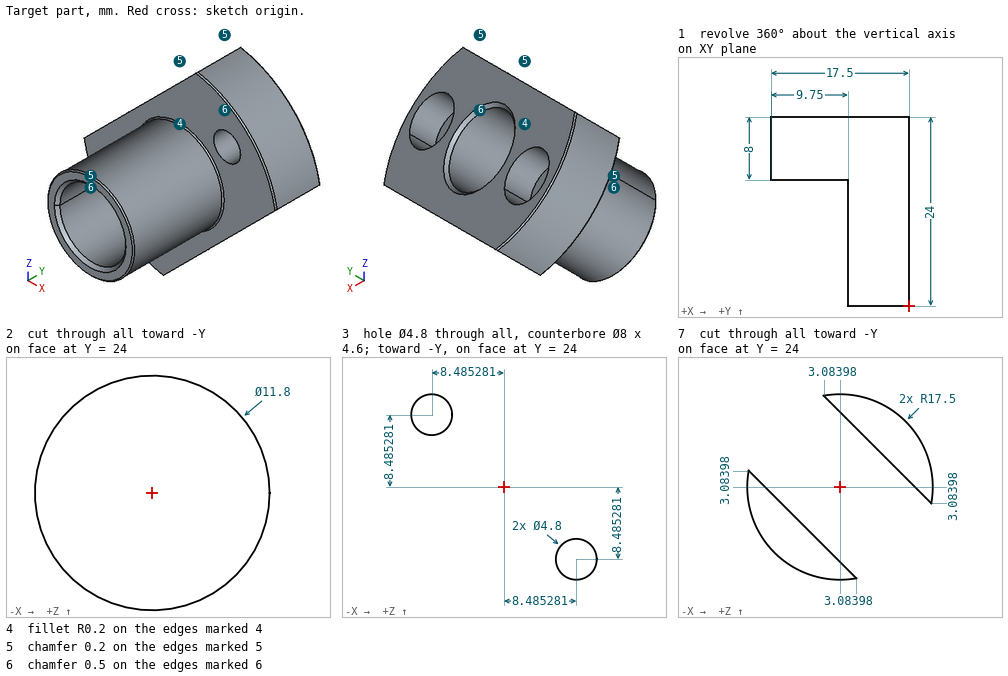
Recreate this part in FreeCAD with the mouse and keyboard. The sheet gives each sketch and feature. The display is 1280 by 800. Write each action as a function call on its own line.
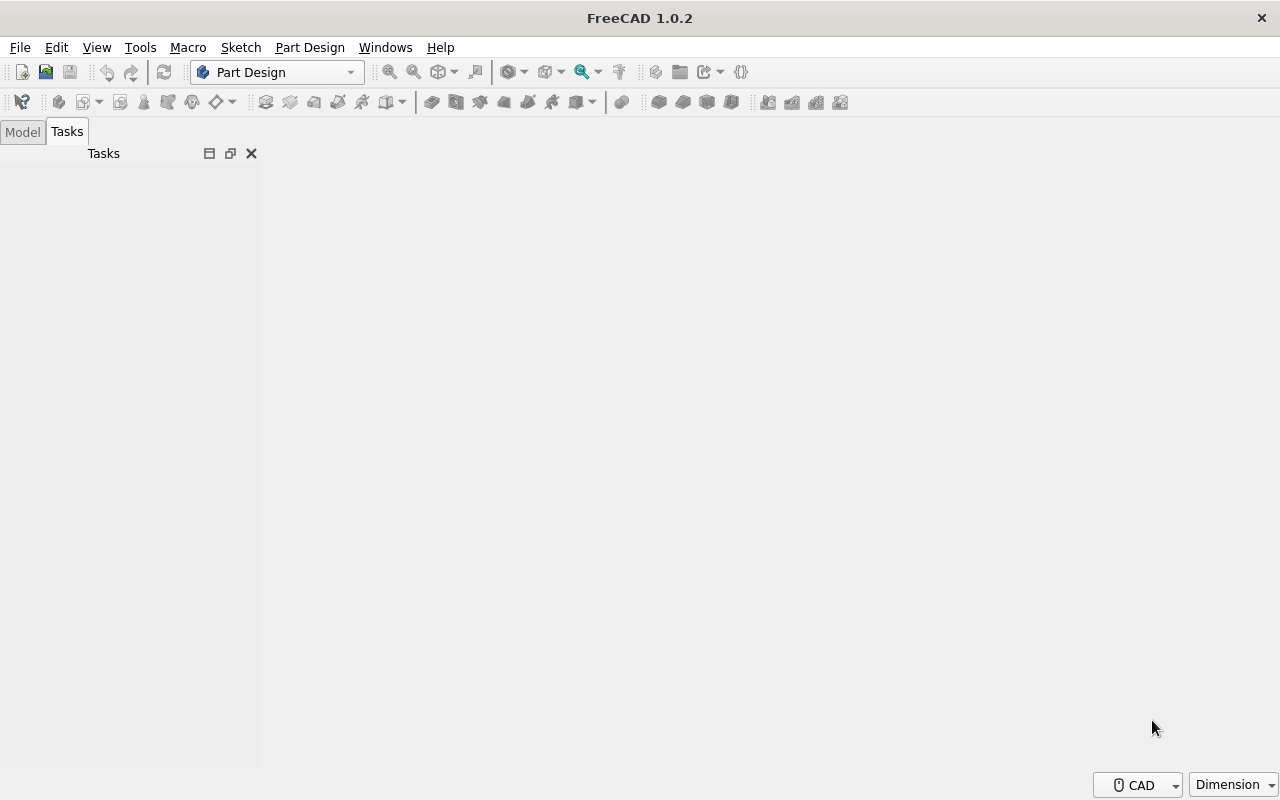
key(ctrl+n)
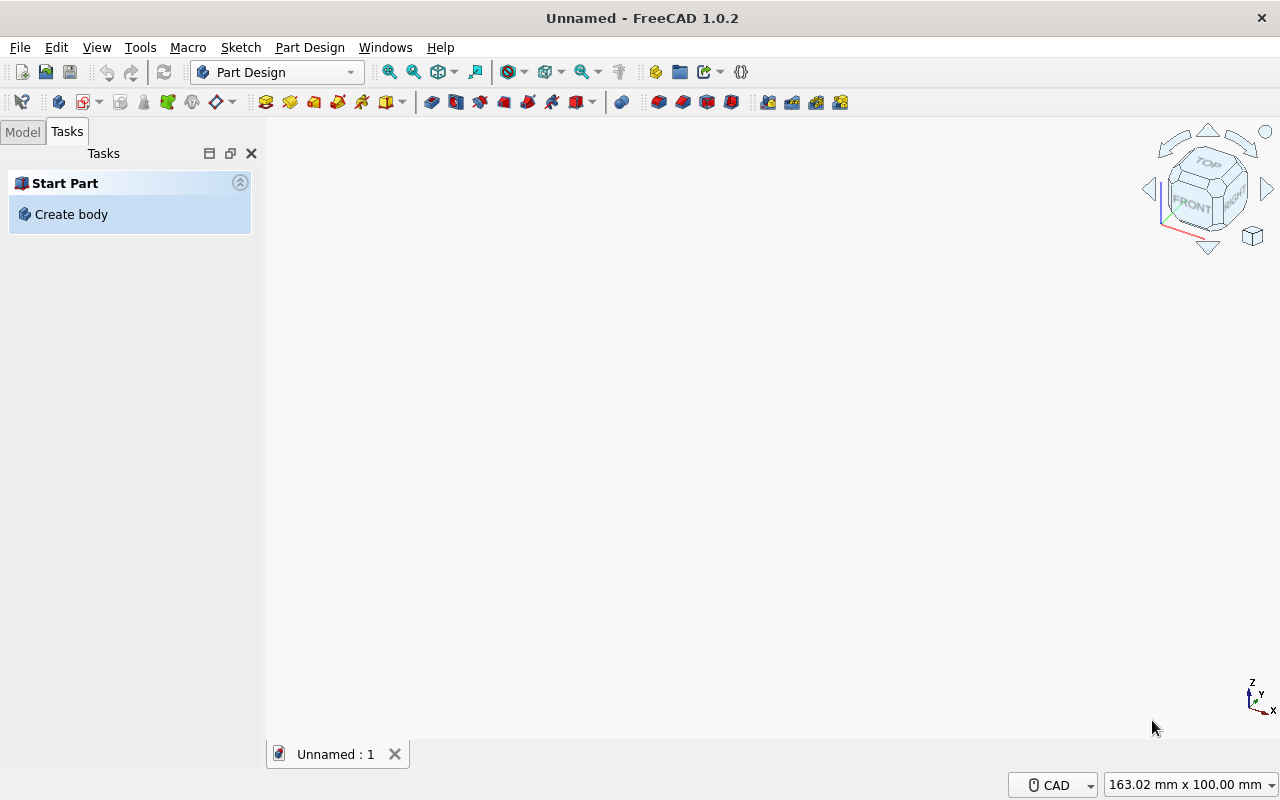
click(84, 102)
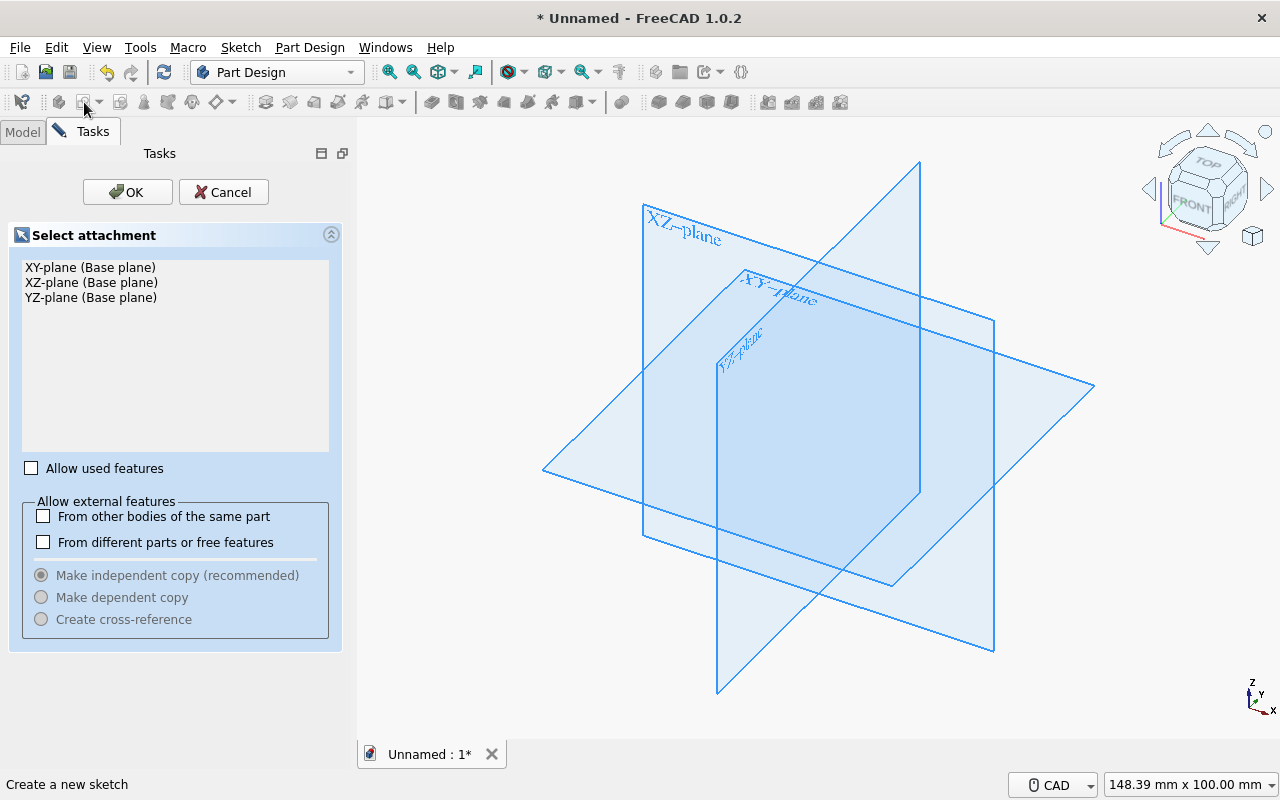
click(82, 268)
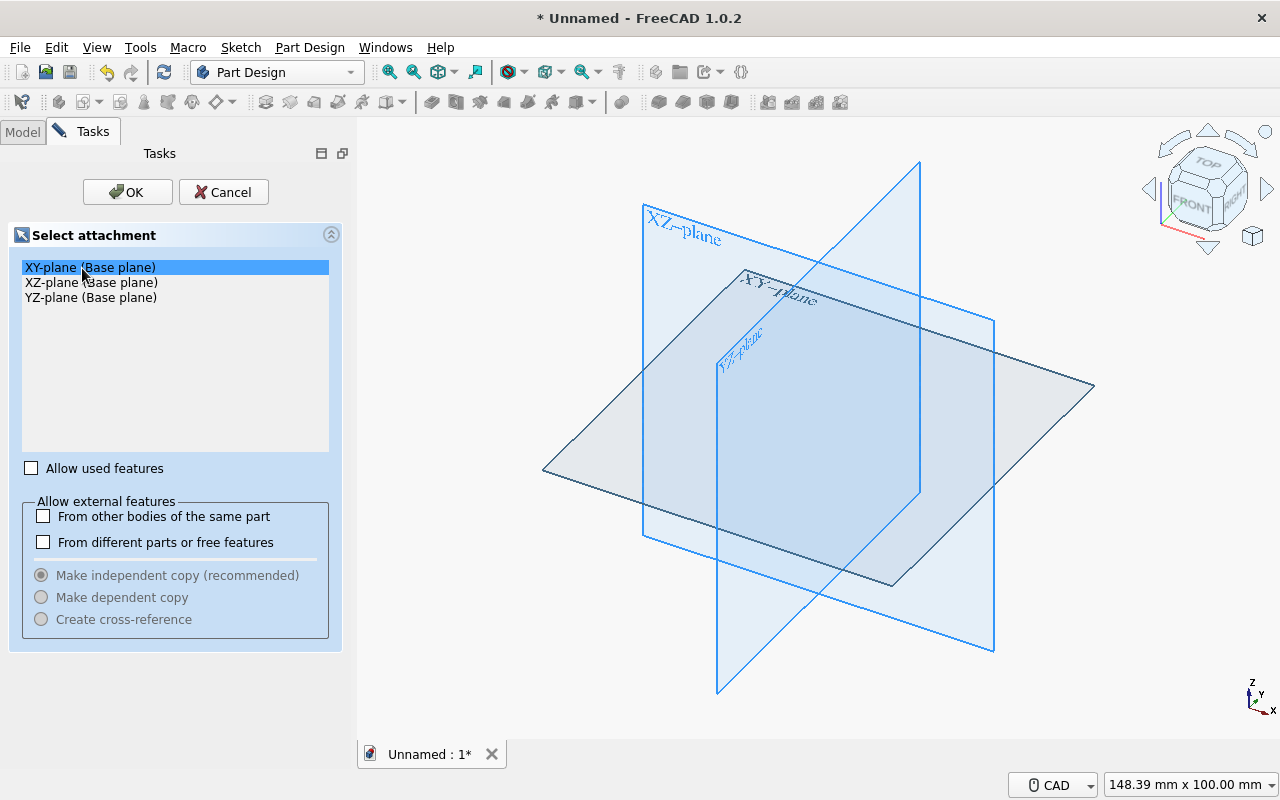
click(128, 192)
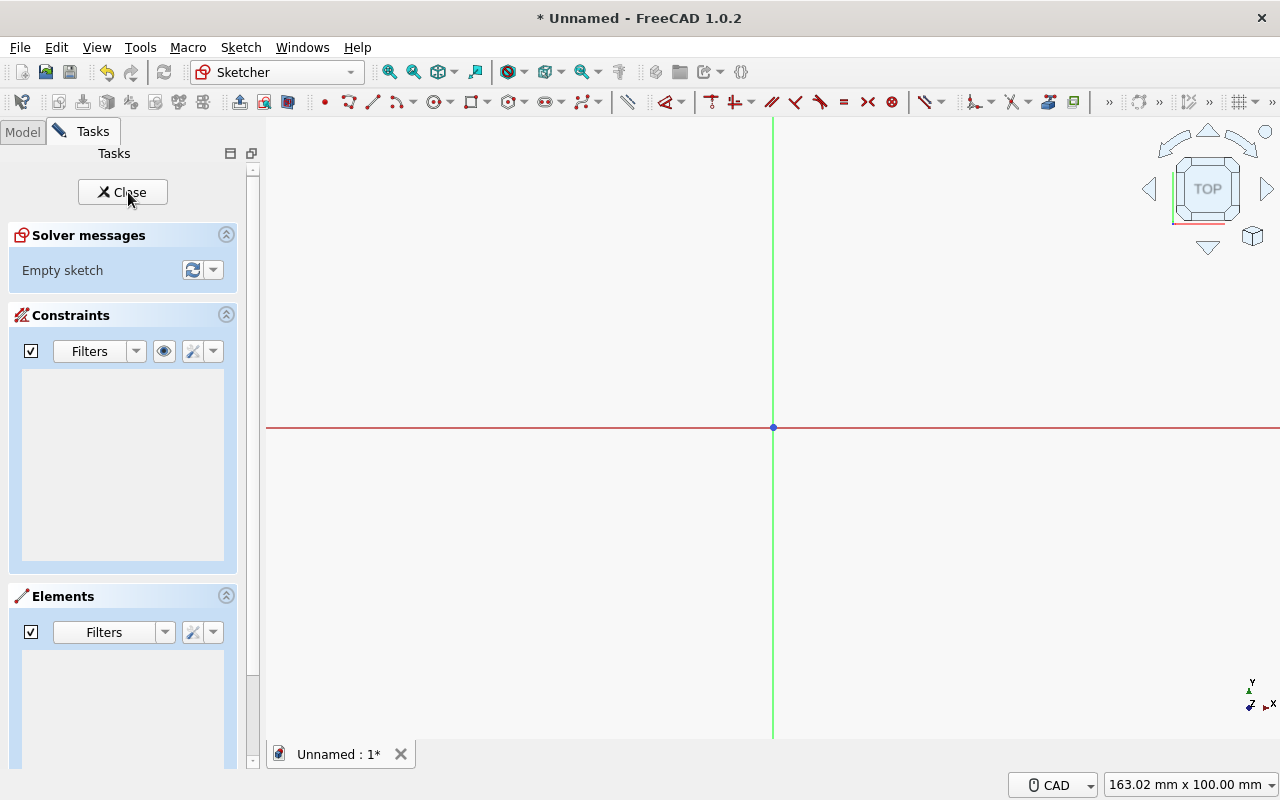
scroll(727, 310, up, 5)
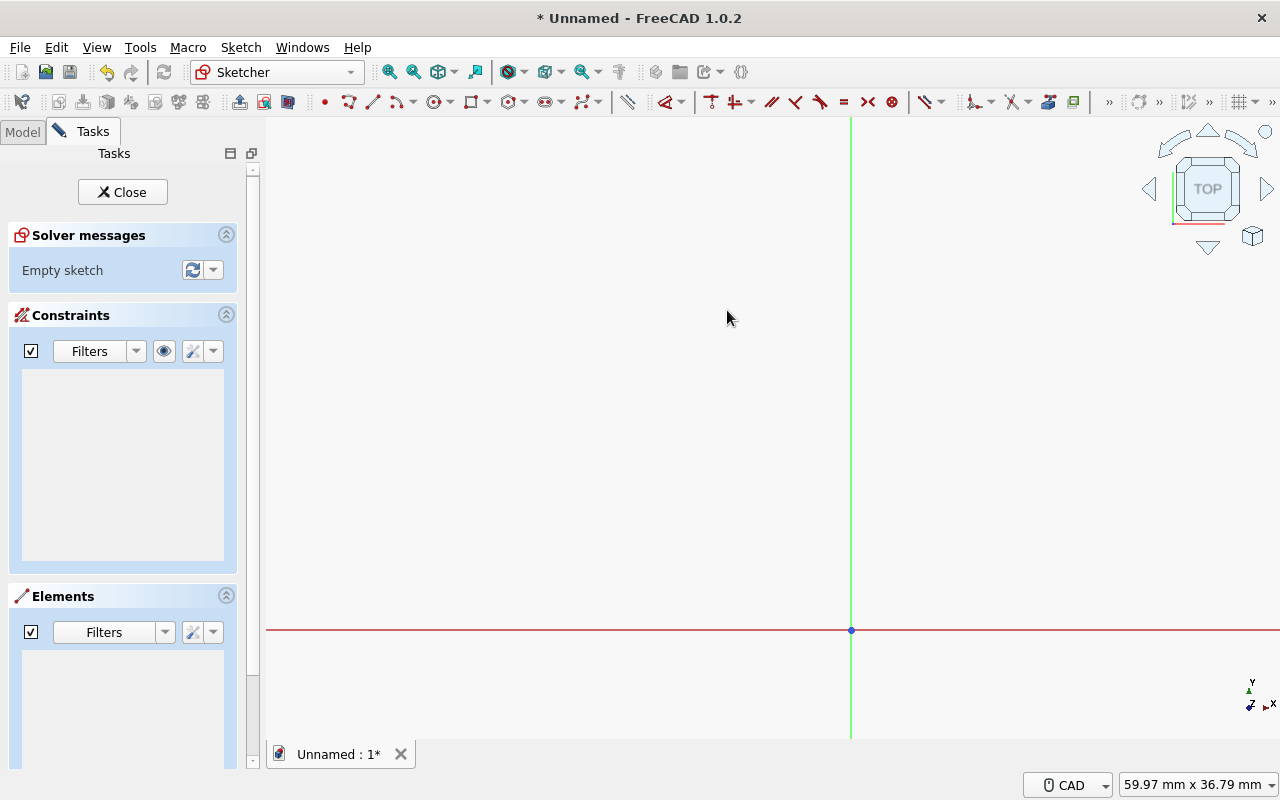
key(g)
key(m)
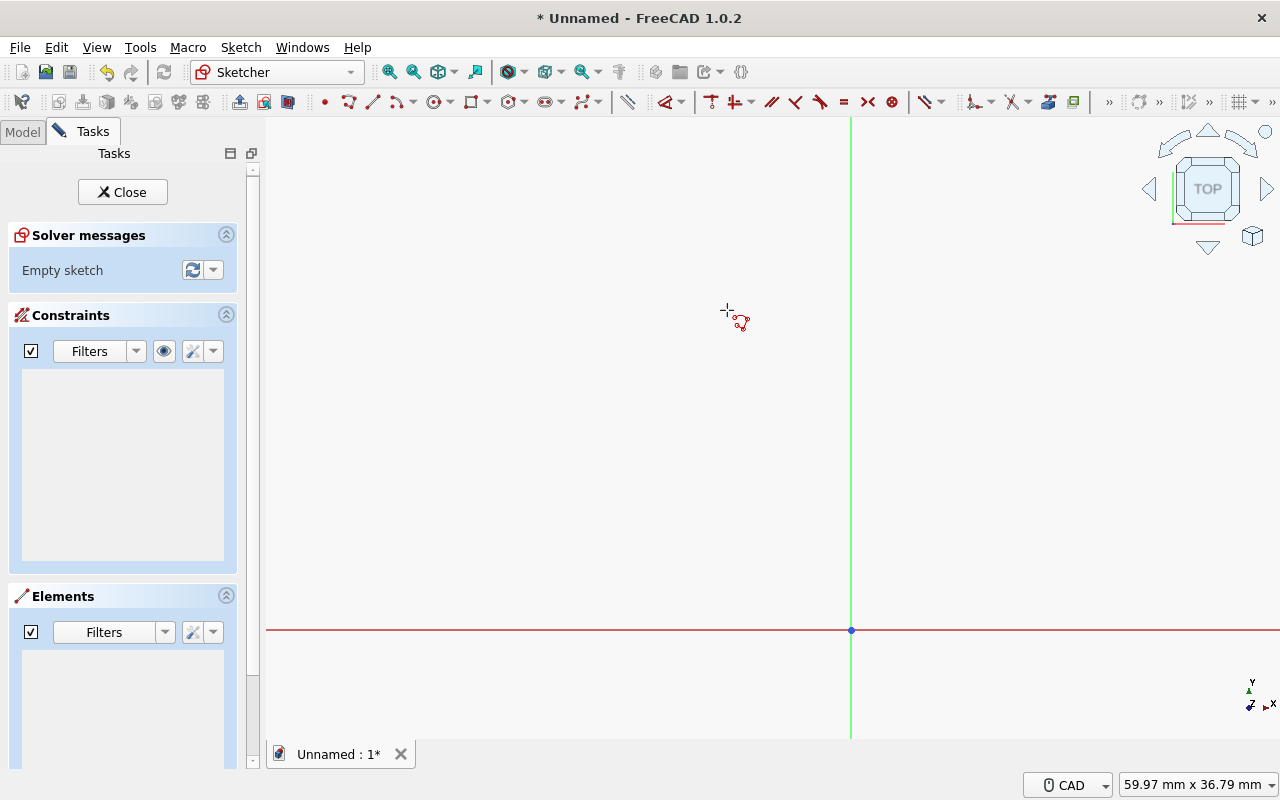
click(851, 630)
click(842, 224)
click(555, 224)
click(555, 360)
click(720, 360)
click(720, 621)
click(851, 630)
key(Escape)
key(Escape)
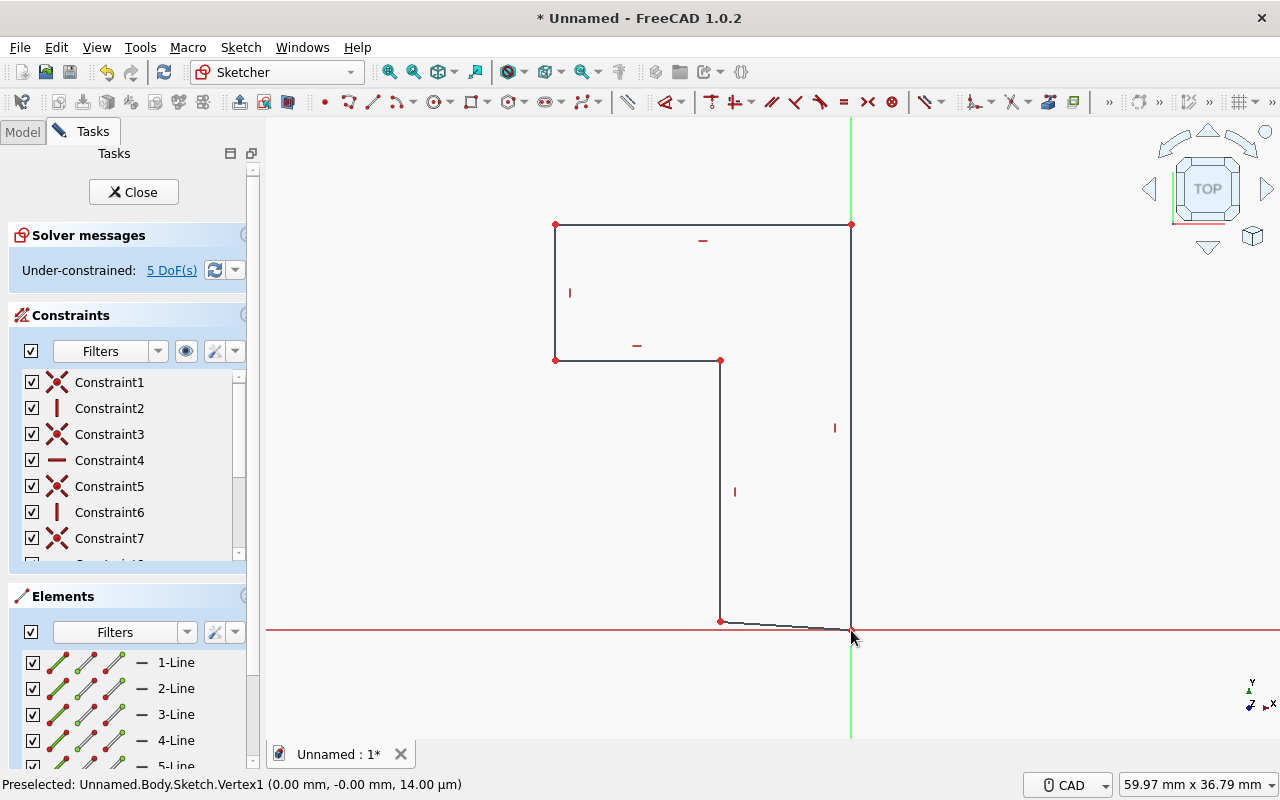
click(812, 628)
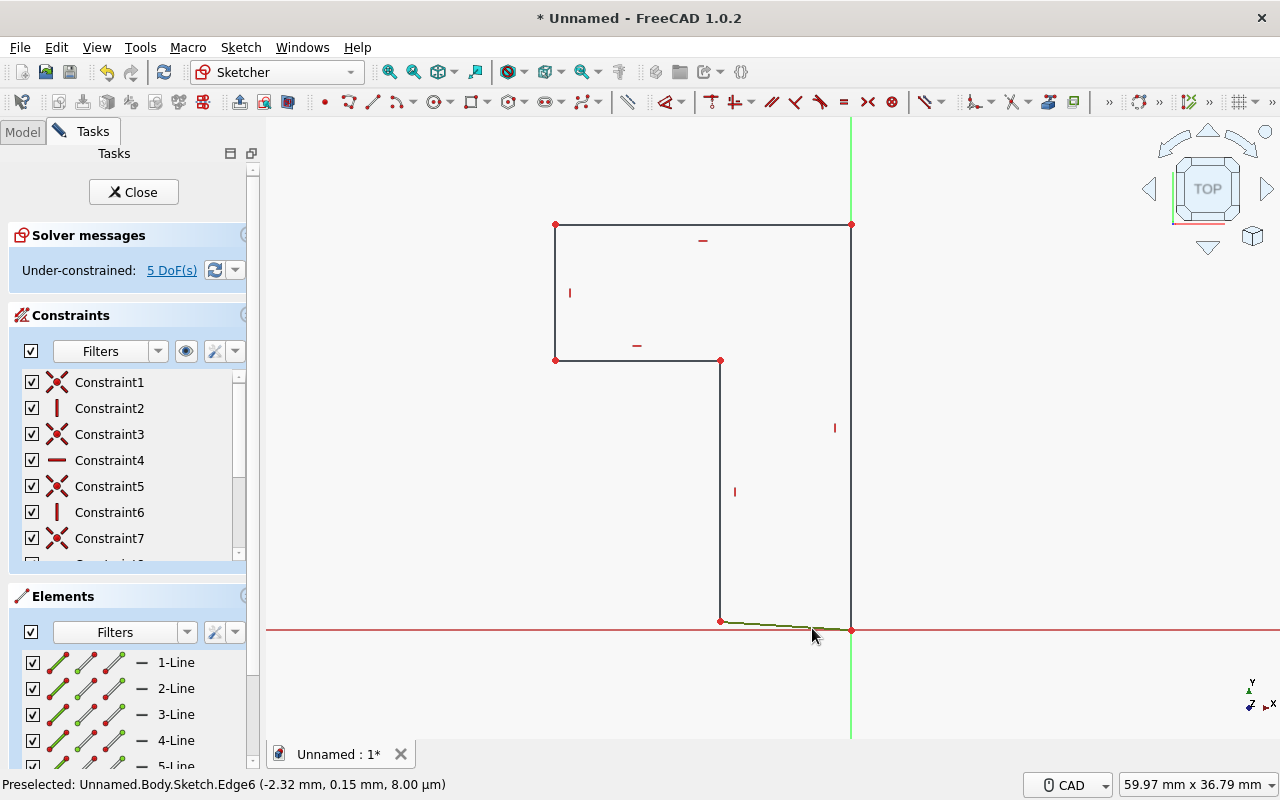
key(h)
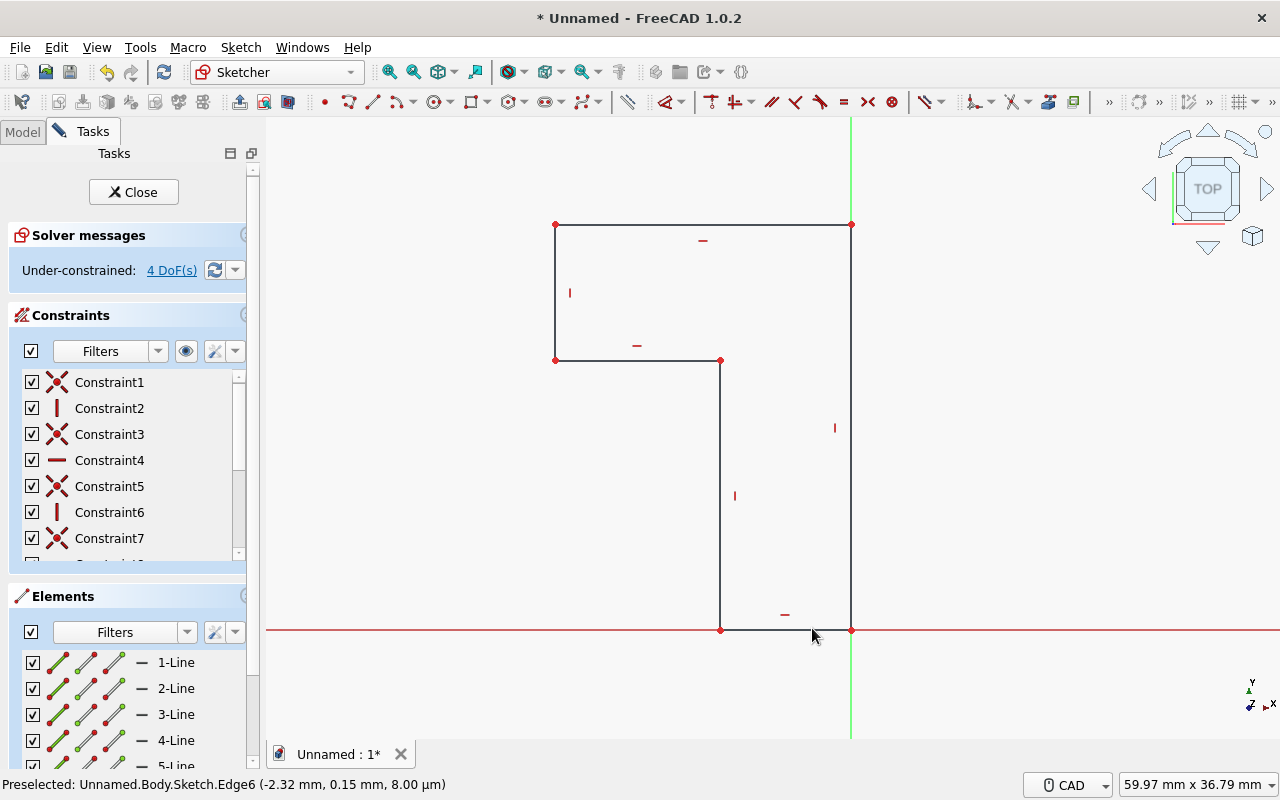
click(555, 266)